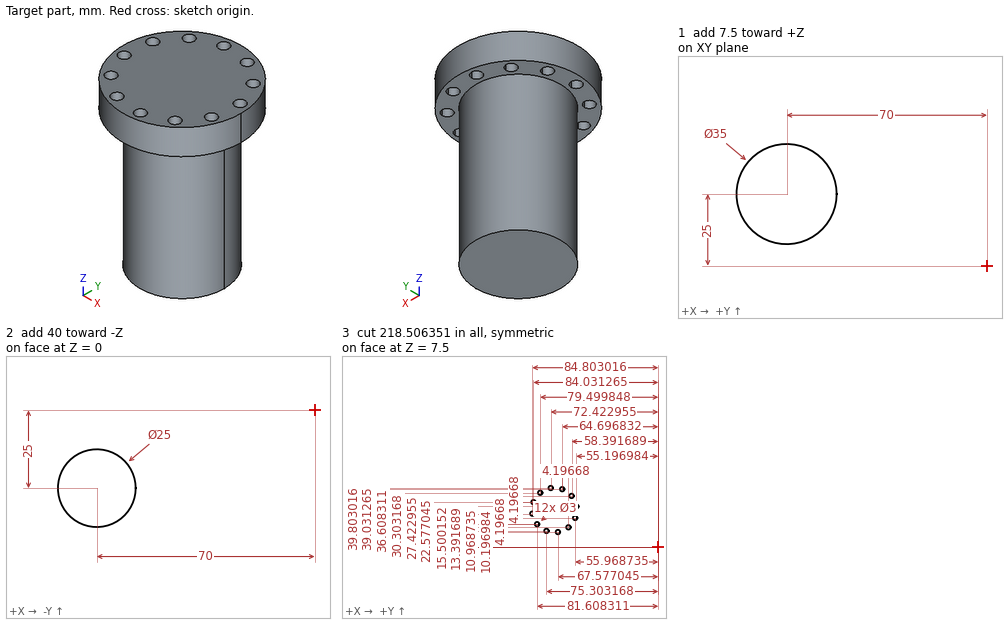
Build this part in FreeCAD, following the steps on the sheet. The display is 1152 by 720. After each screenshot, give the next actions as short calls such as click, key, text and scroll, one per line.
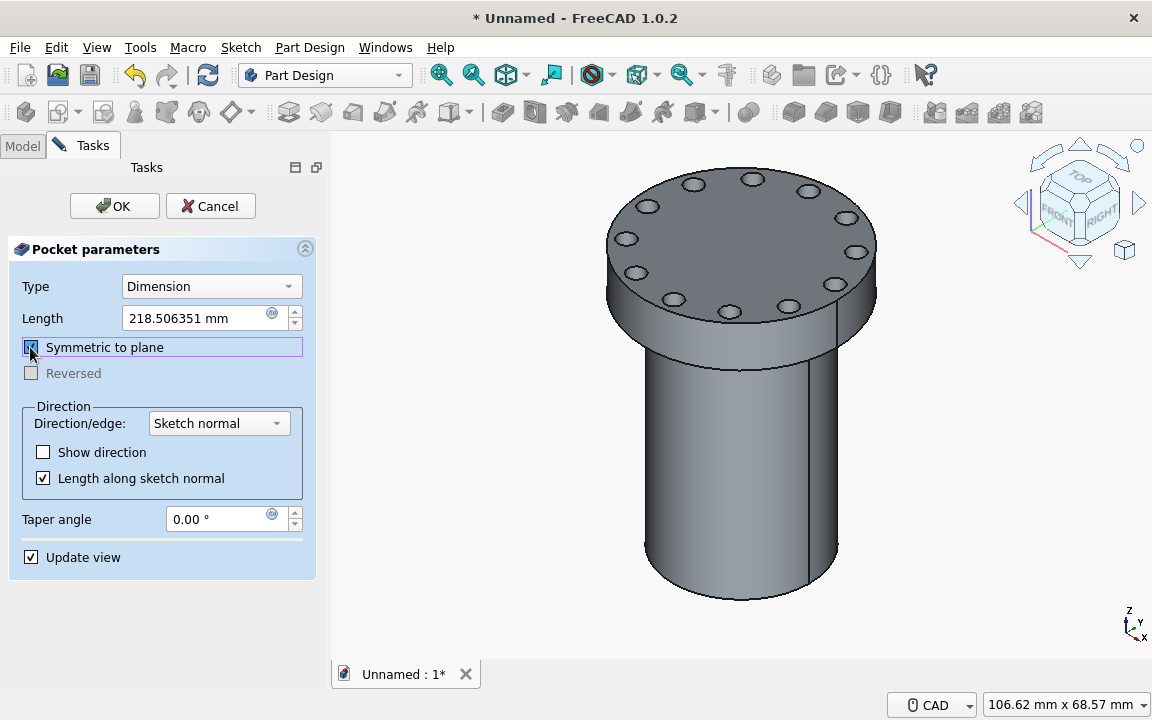
click(115, 206)